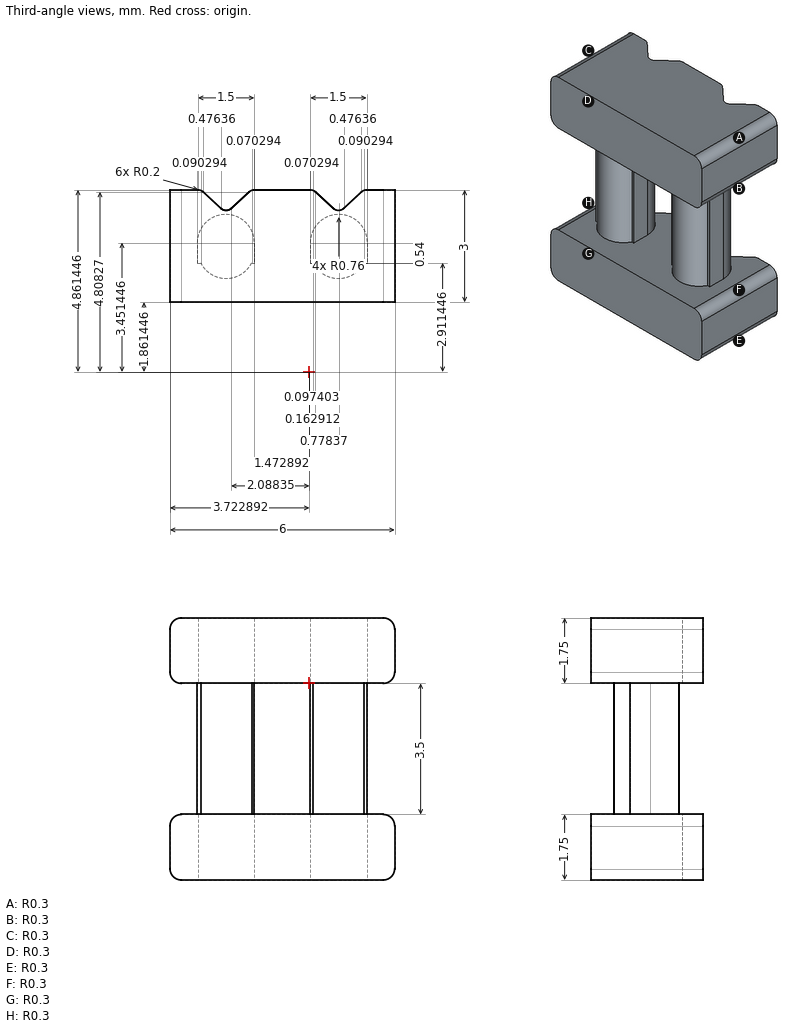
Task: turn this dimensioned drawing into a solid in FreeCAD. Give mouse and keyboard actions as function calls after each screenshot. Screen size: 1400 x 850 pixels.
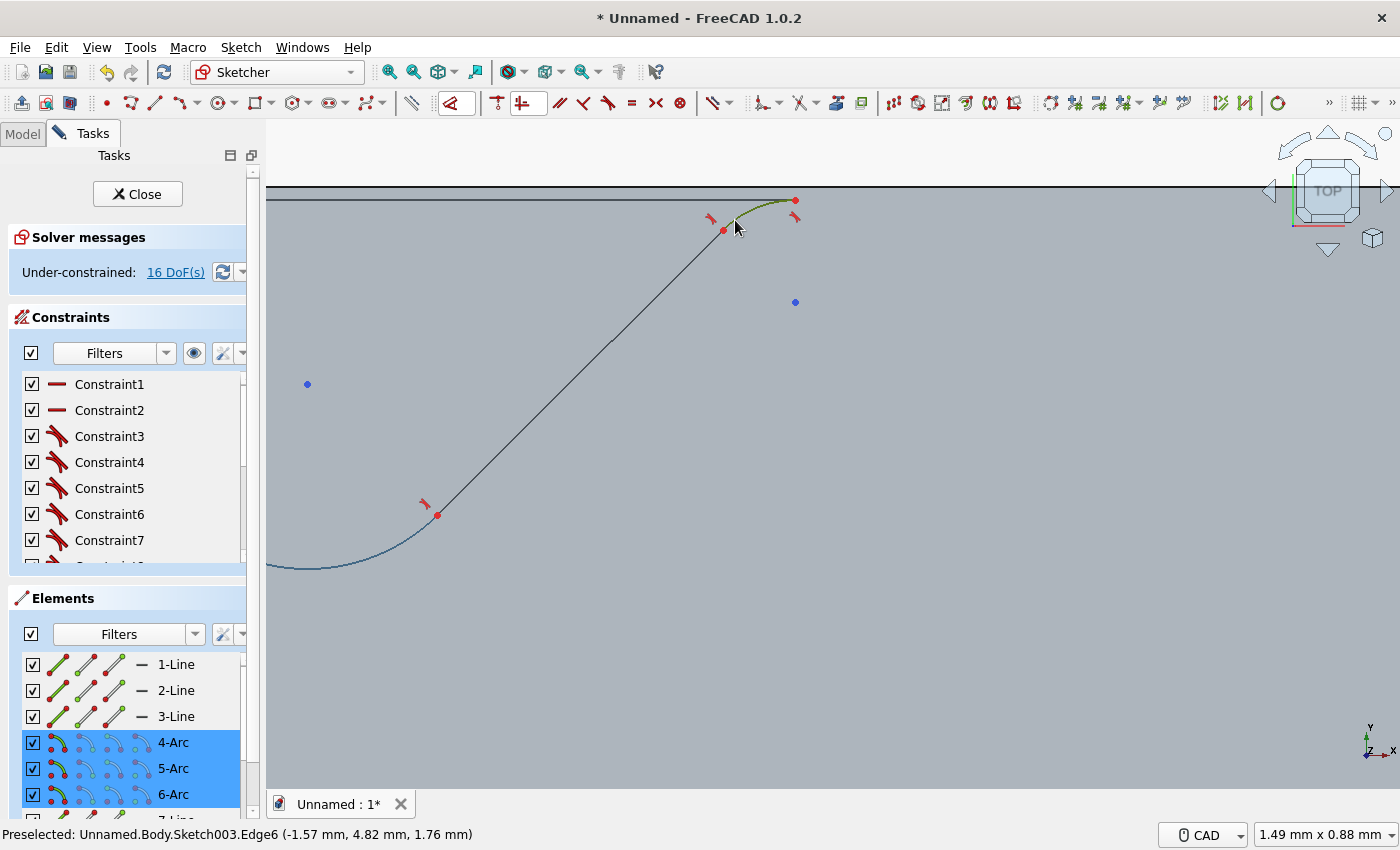
scroll(687, 257, down, 11)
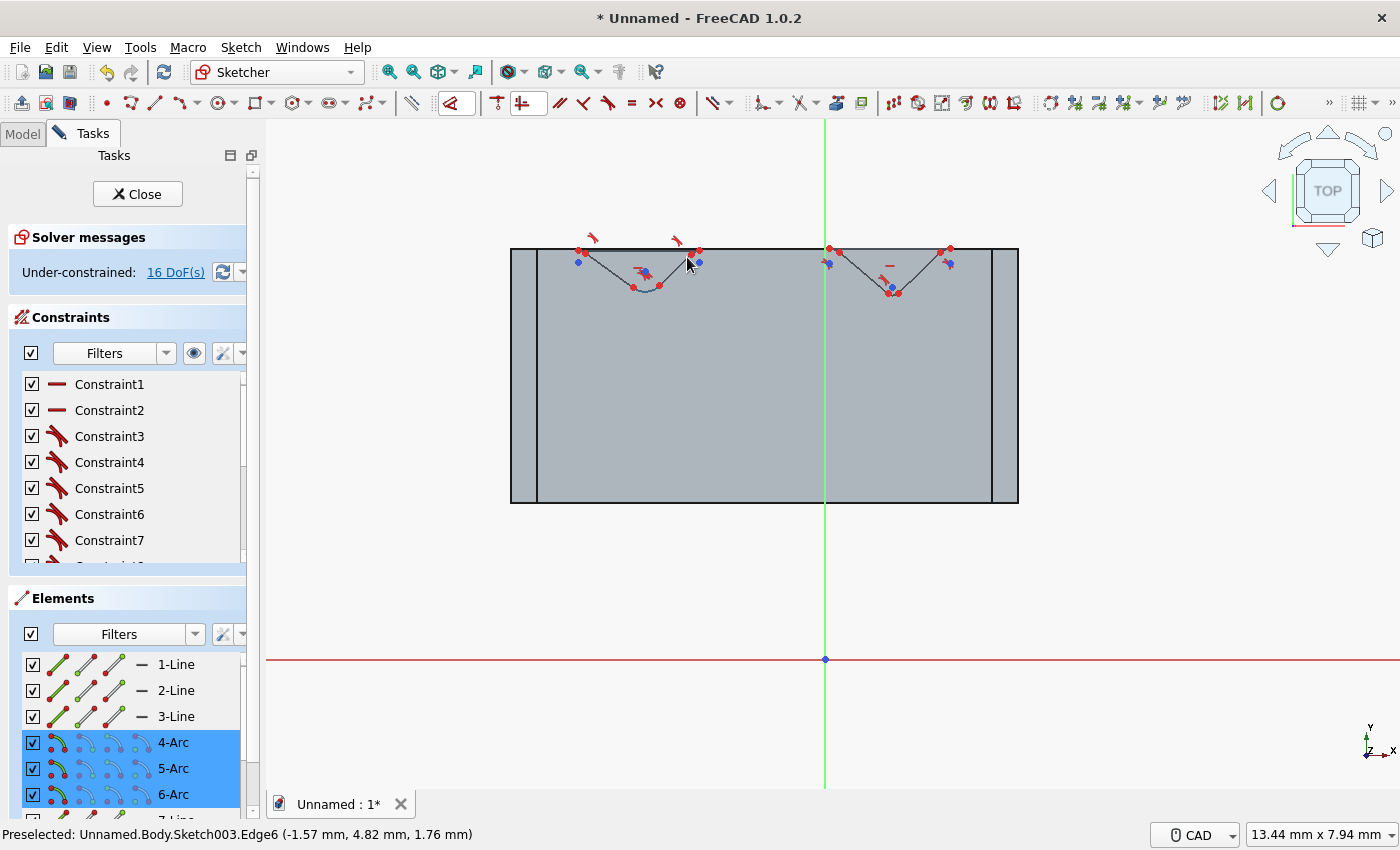
scroll(891, 295, up, 8)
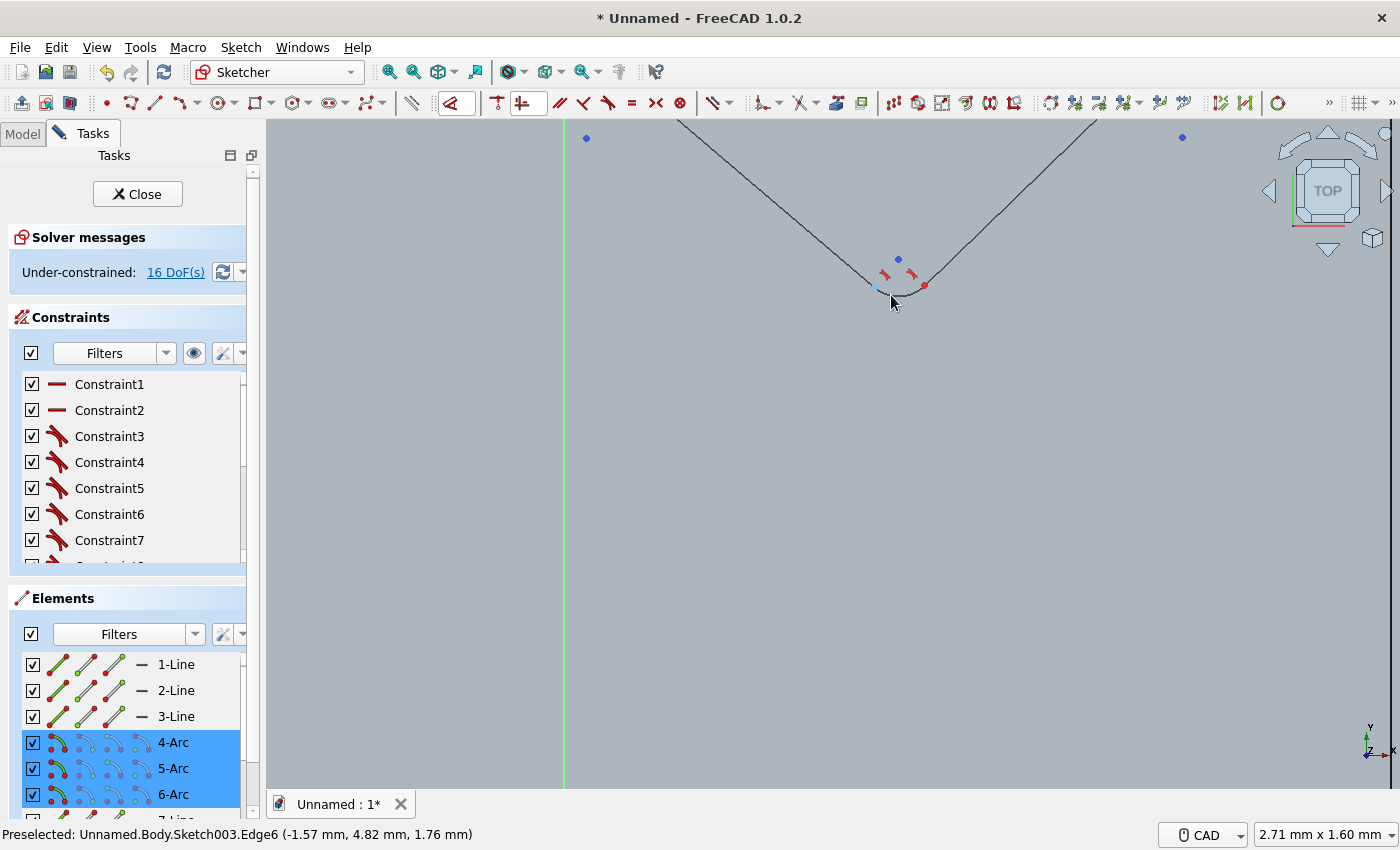
click(889, 295)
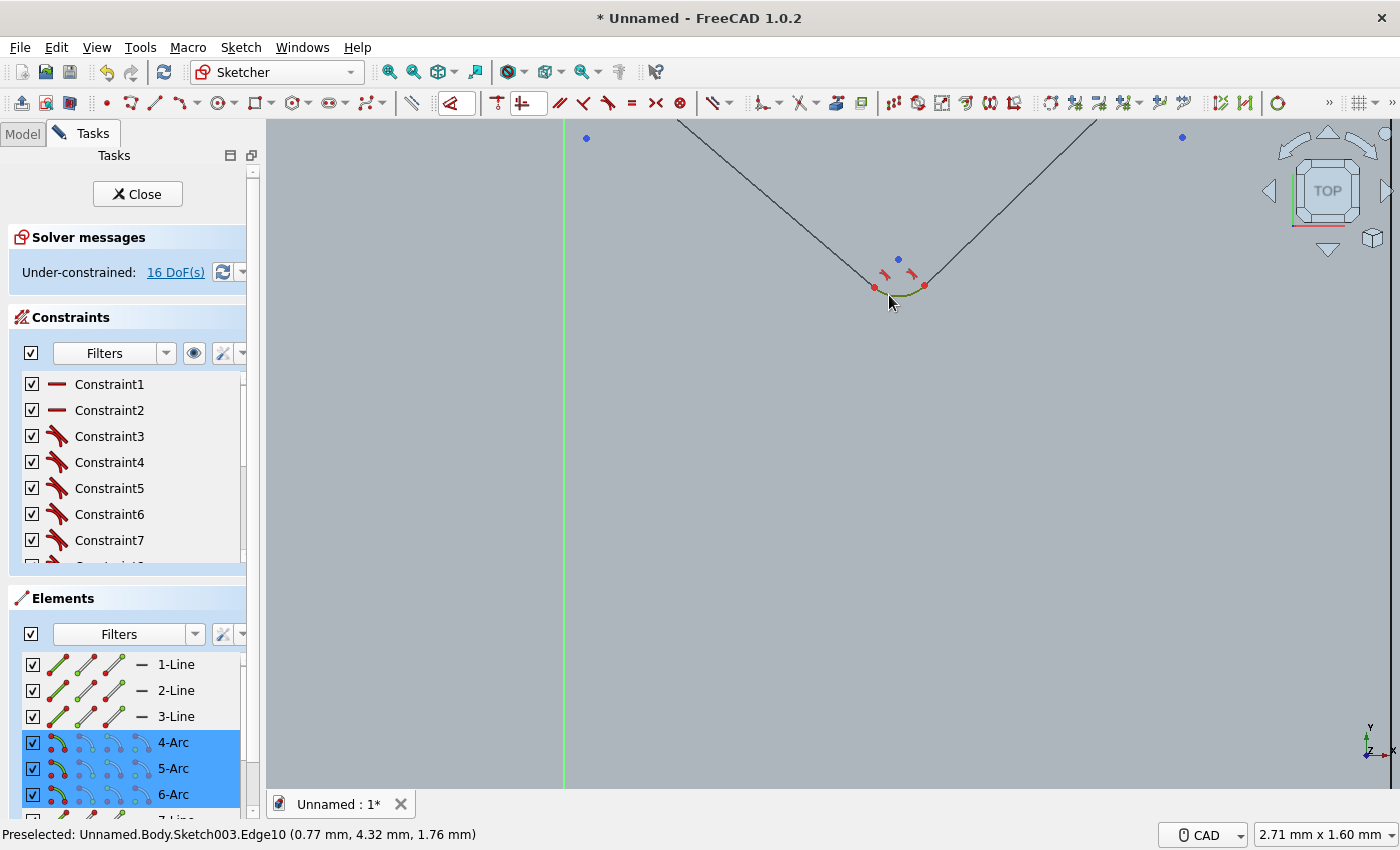
scroll(892, 295, down, 8)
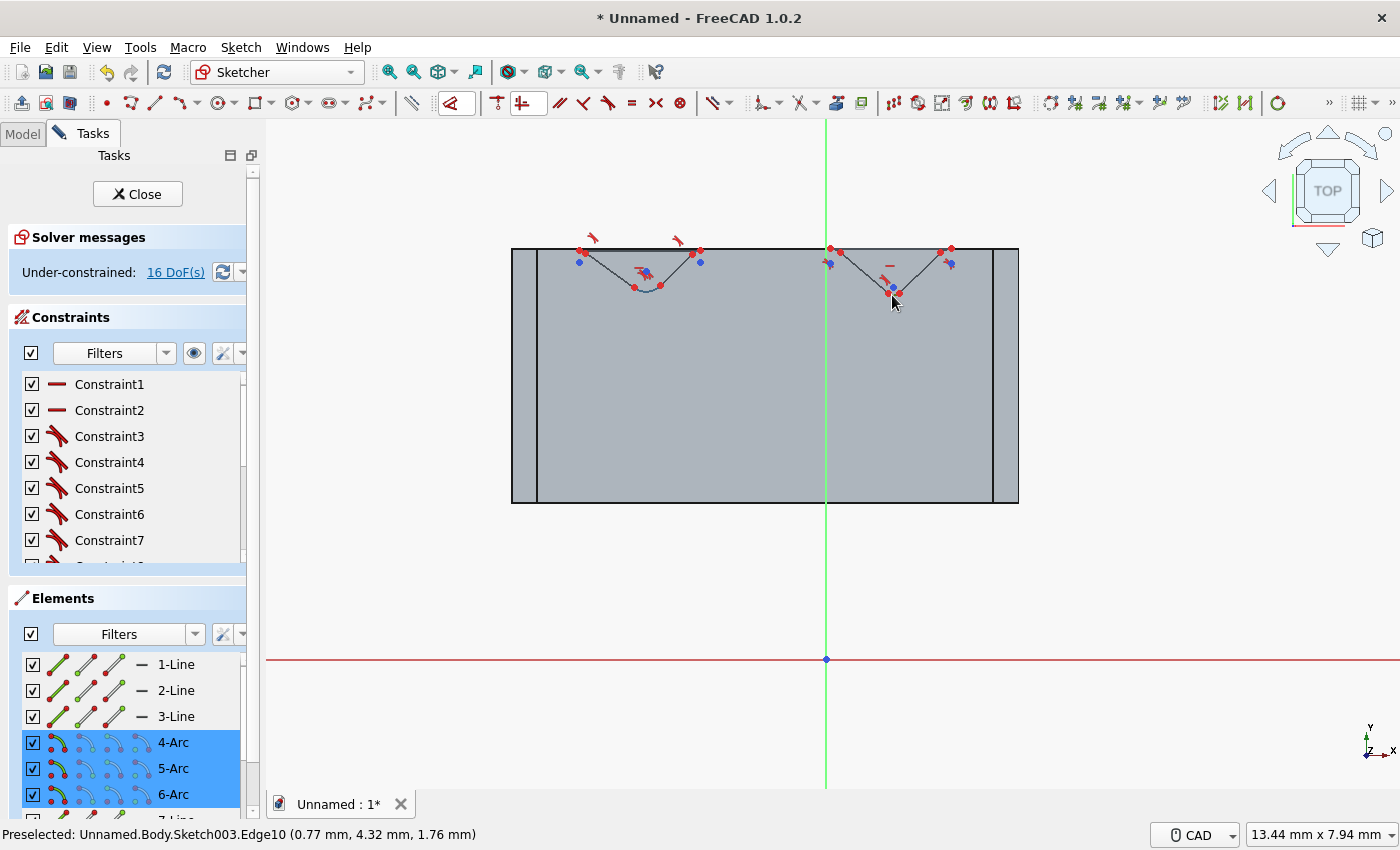
scroll(944, 251, up, 10)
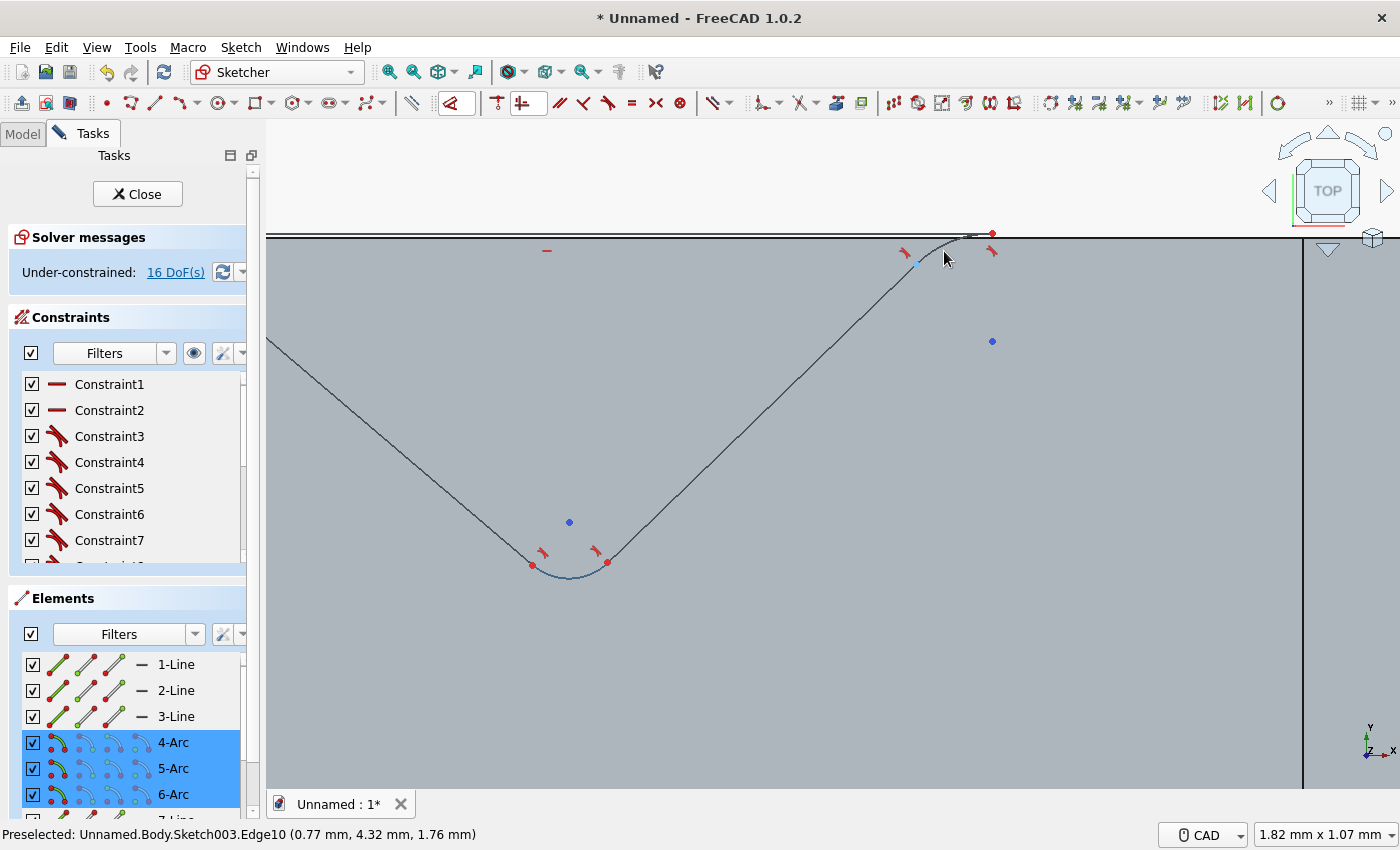
click(937, 249)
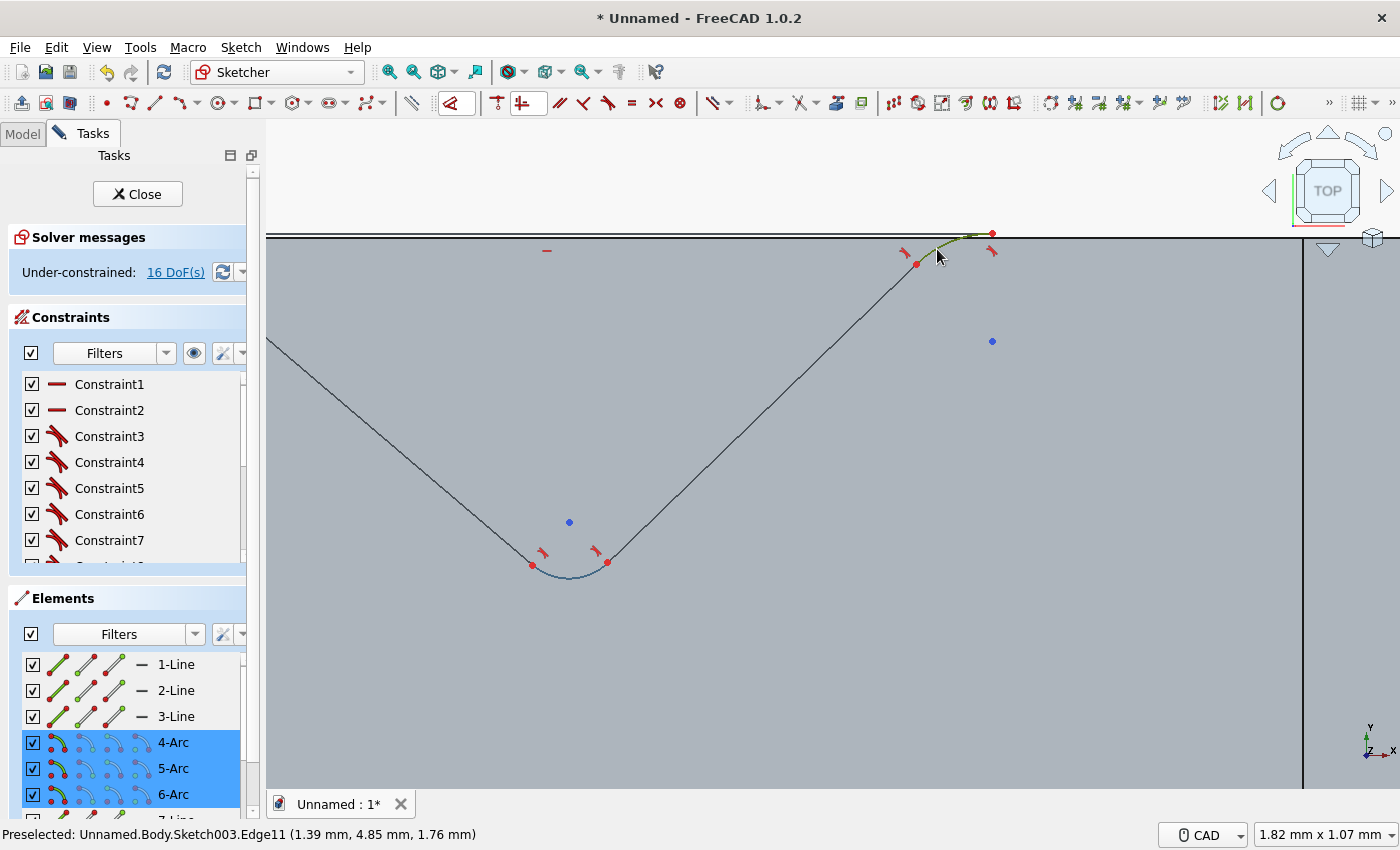
scroll(944, 251, down, 10)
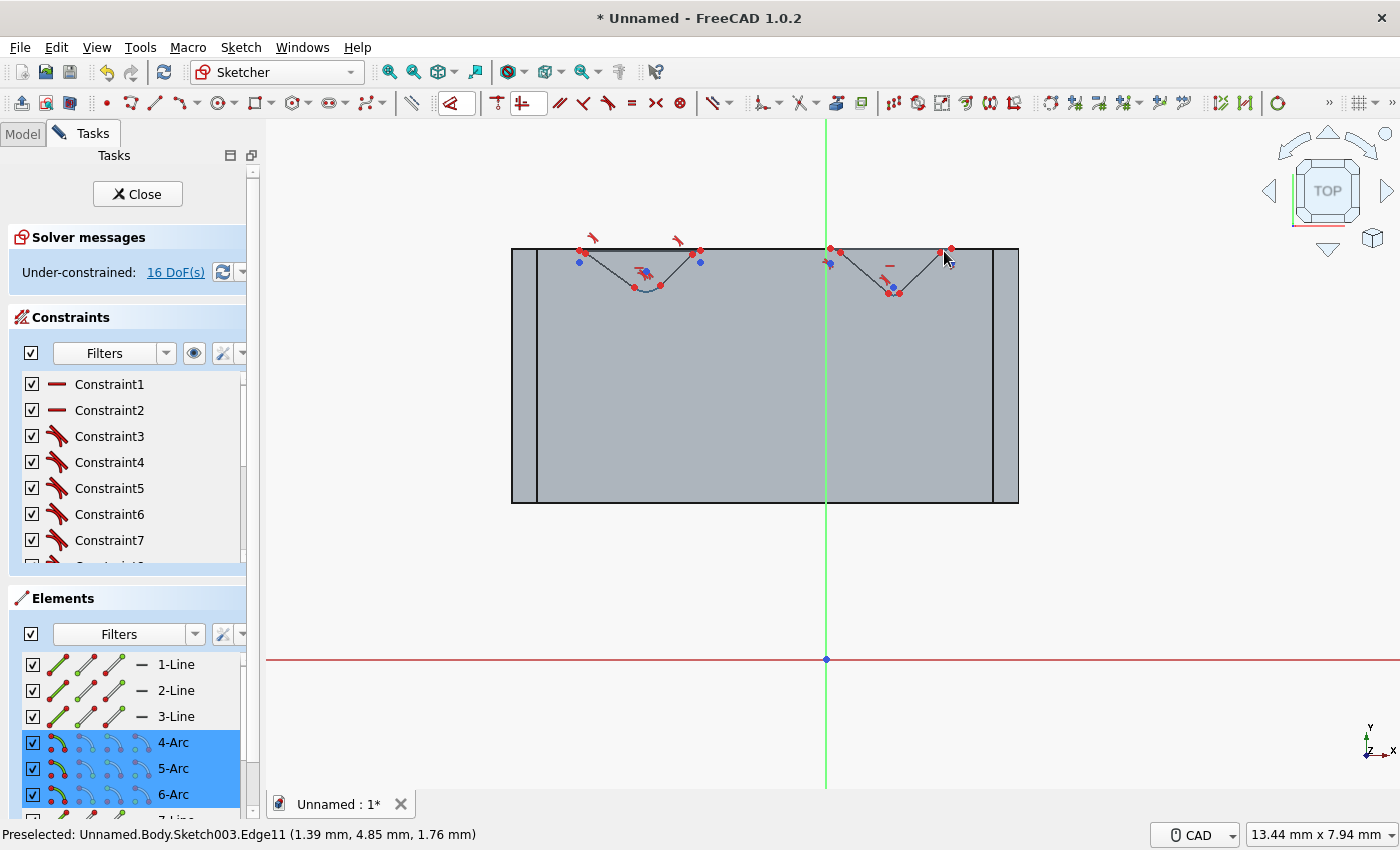
scroll(838, 251, up, 11)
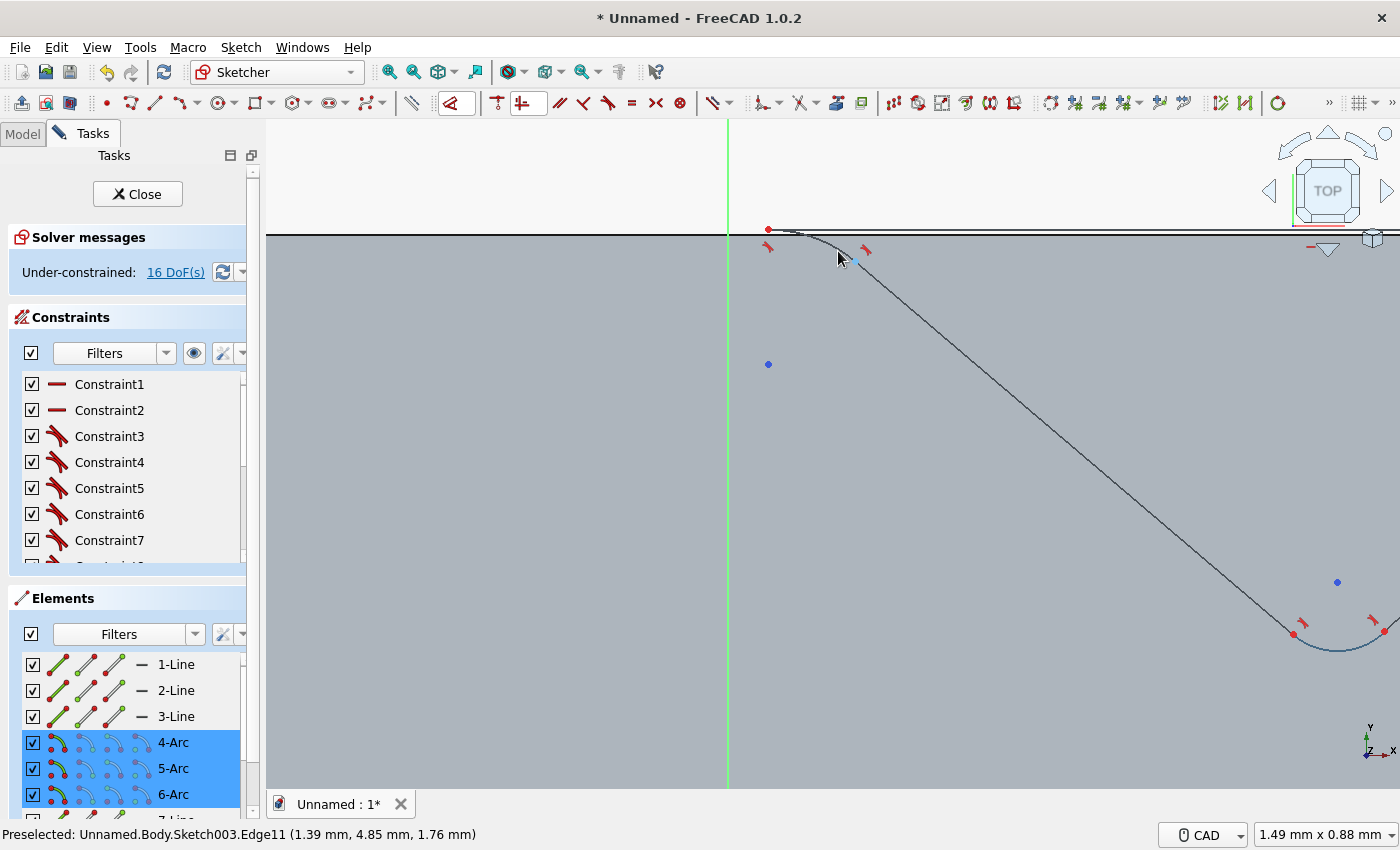
click(832, 246)